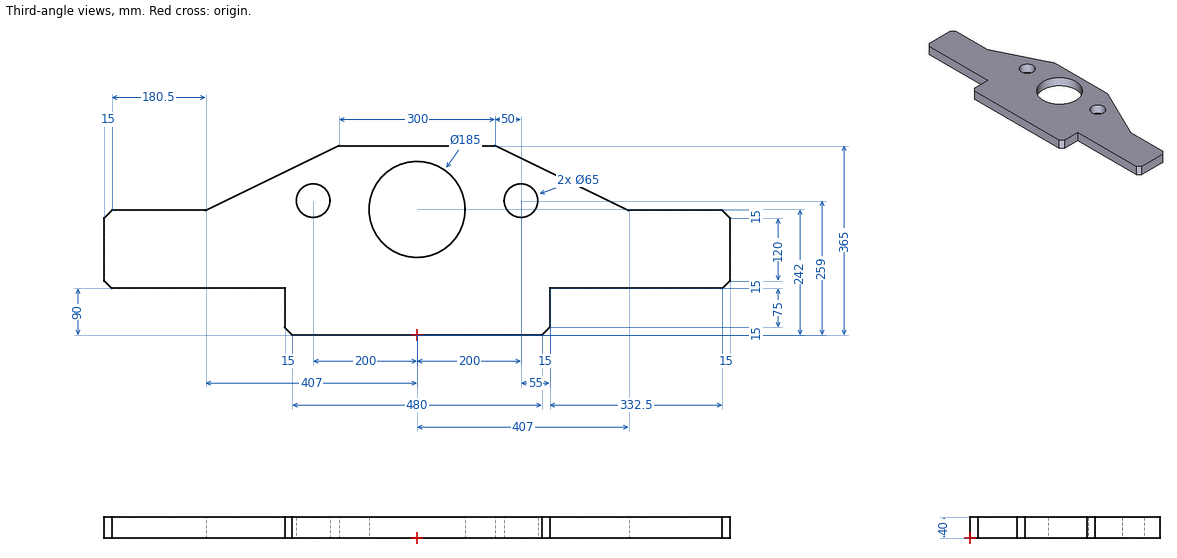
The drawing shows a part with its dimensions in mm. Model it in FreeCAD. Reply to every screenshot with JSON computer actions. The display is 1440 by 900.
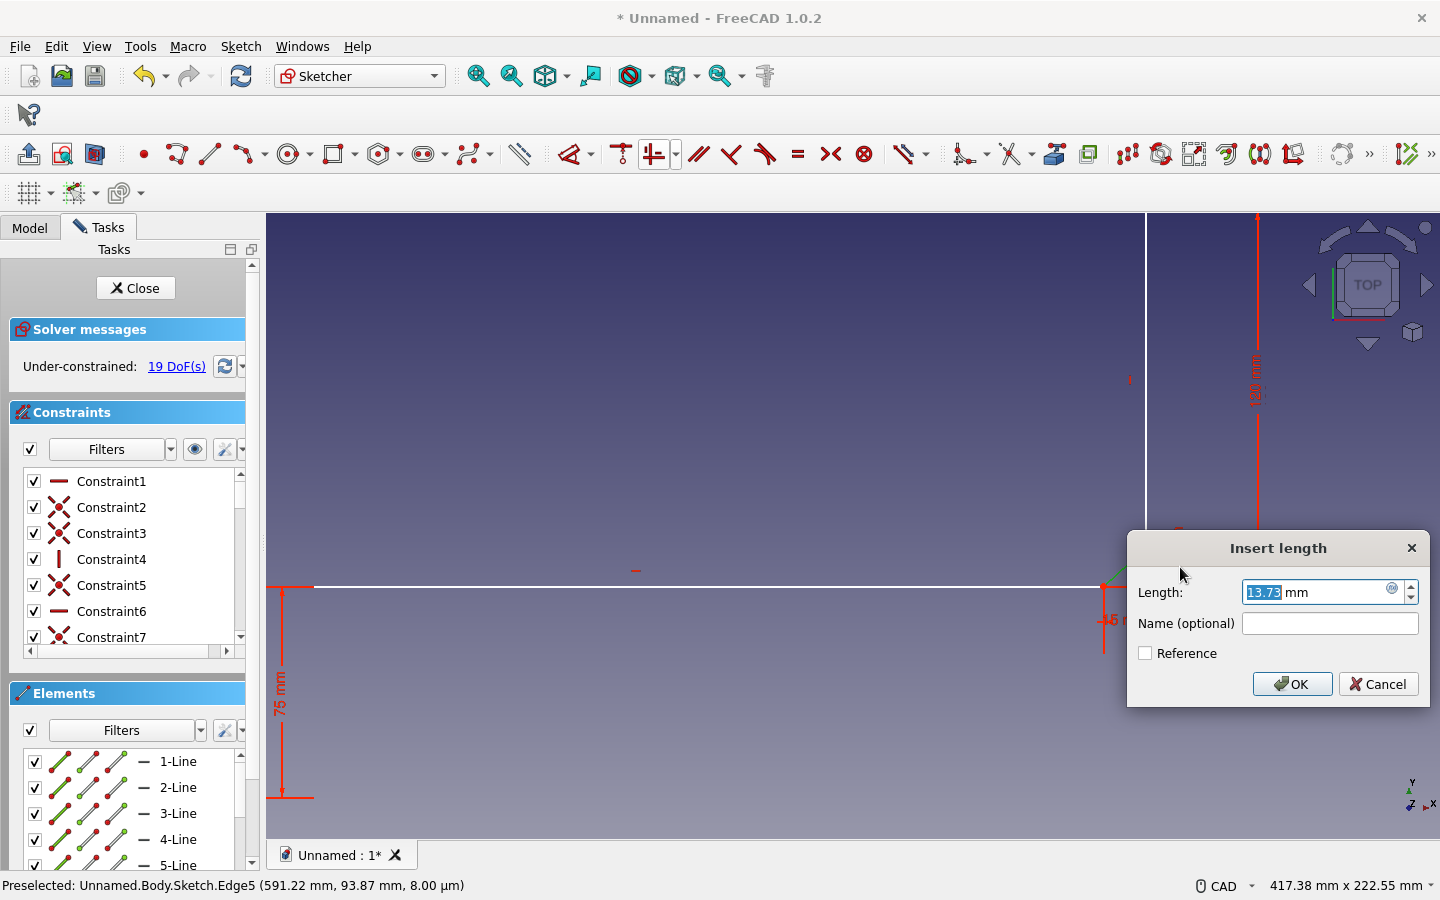
{"action": "type", "text": "15"}
{"action": "key", "text": "Return"}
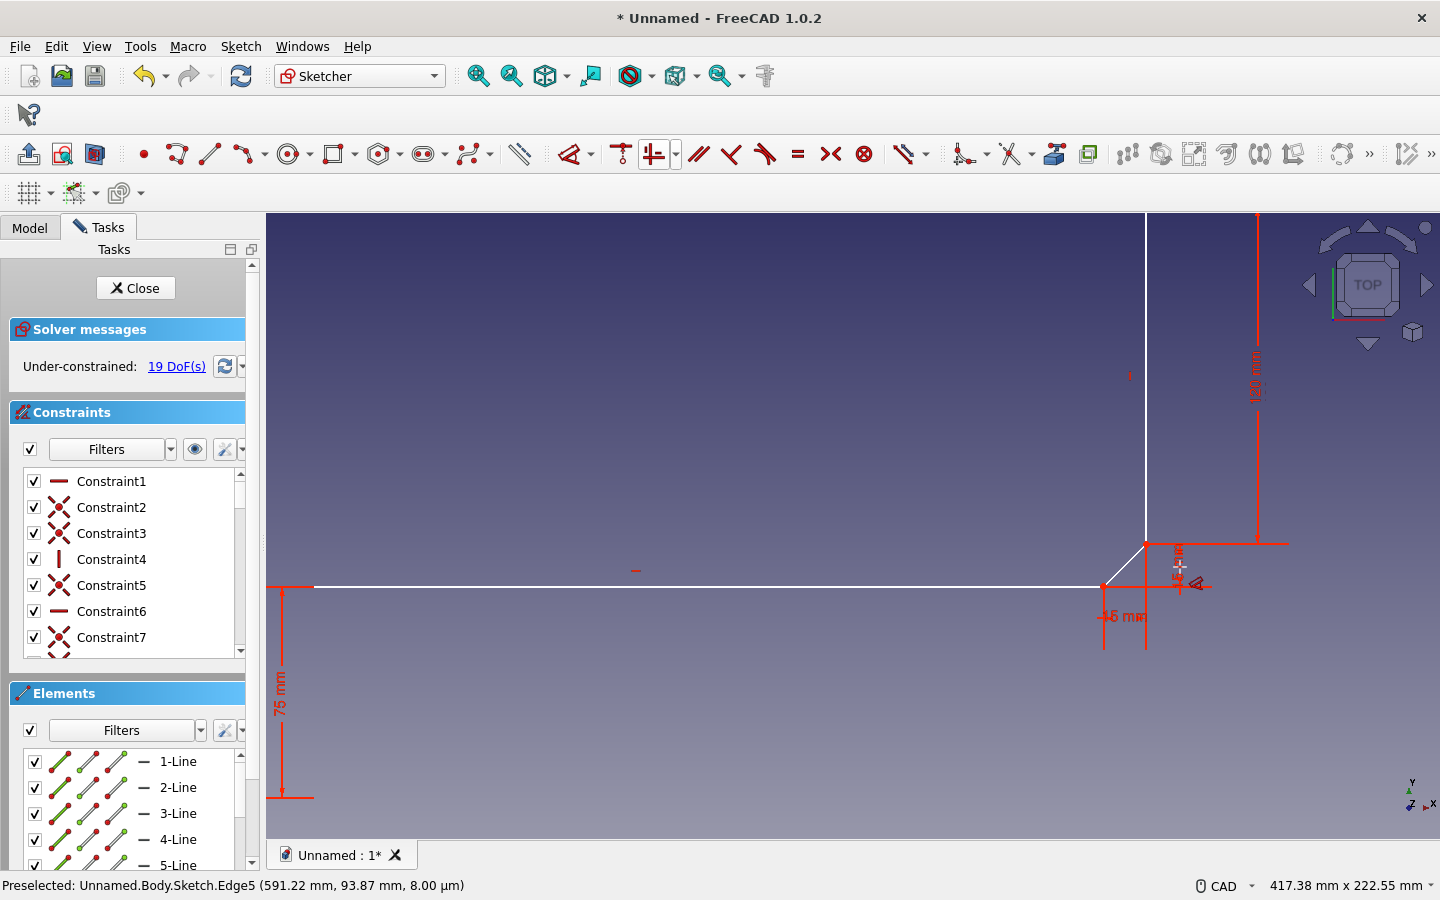
{"action": "scroll", "coordinate": [1121, 576], "scroll_direction": "down", "scroll_amount": 8}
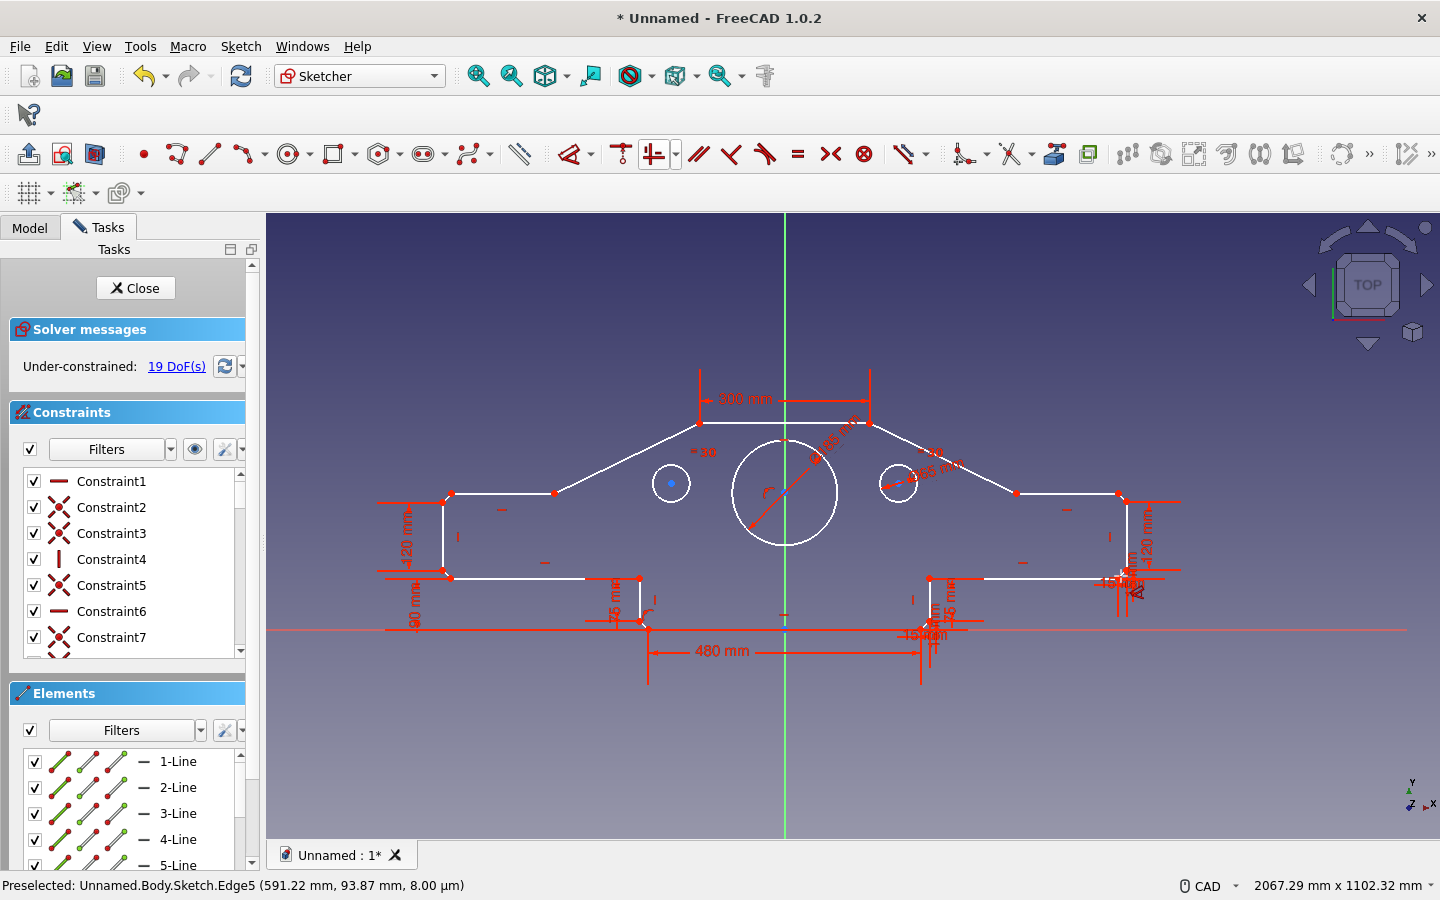
{"action": "scroll", "coordinate": [1124, 499], "scroll_direction": "up", "scroll_amount": 8}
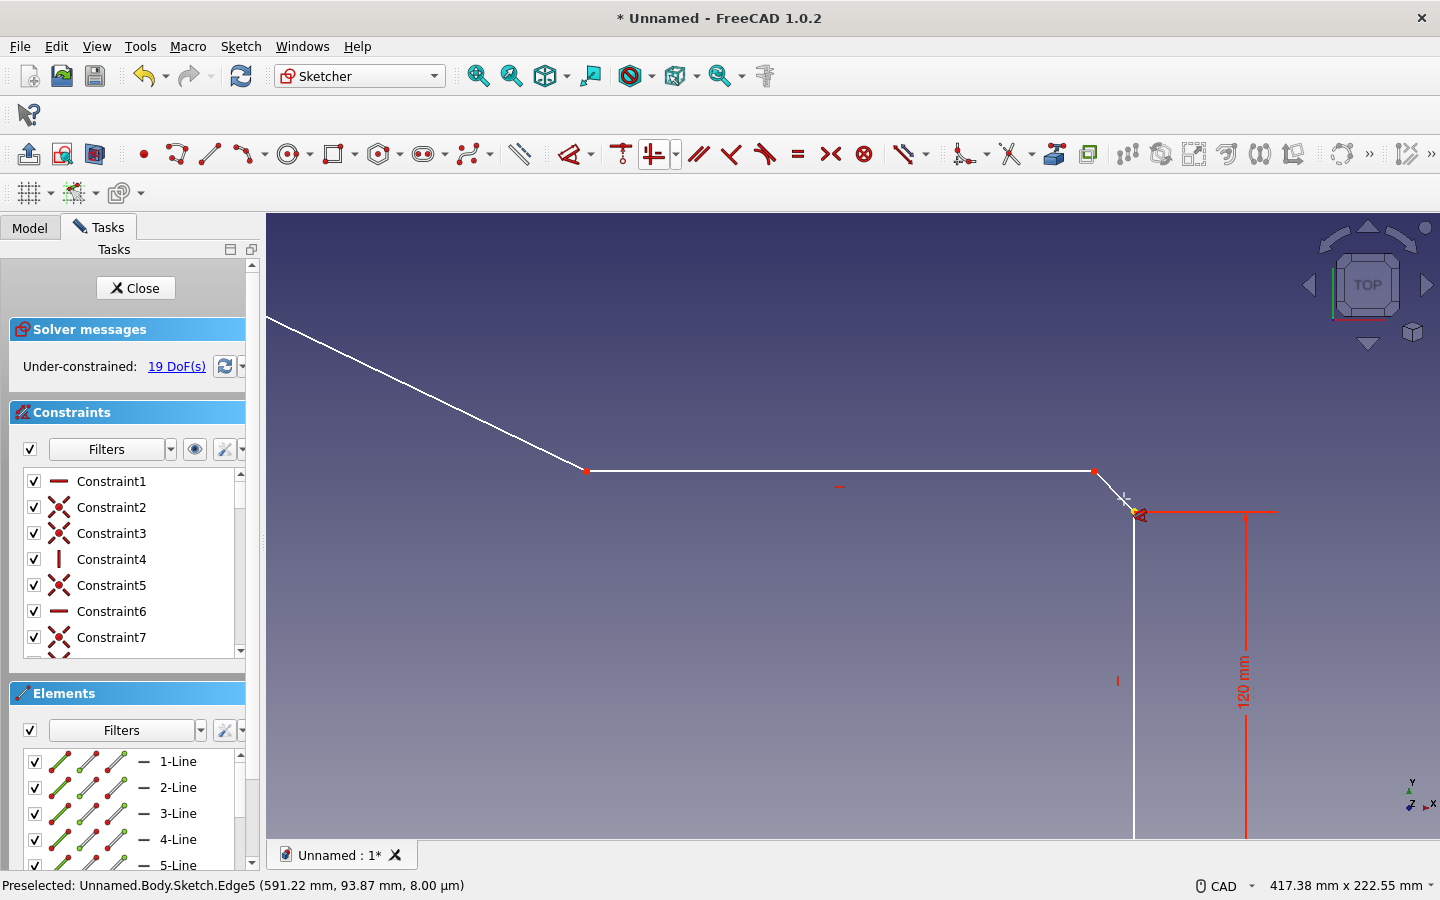
{"action": "left_click", "coordinate": [1122, 500]}
{"action": "left_click", "coordinate": [1114, 437]}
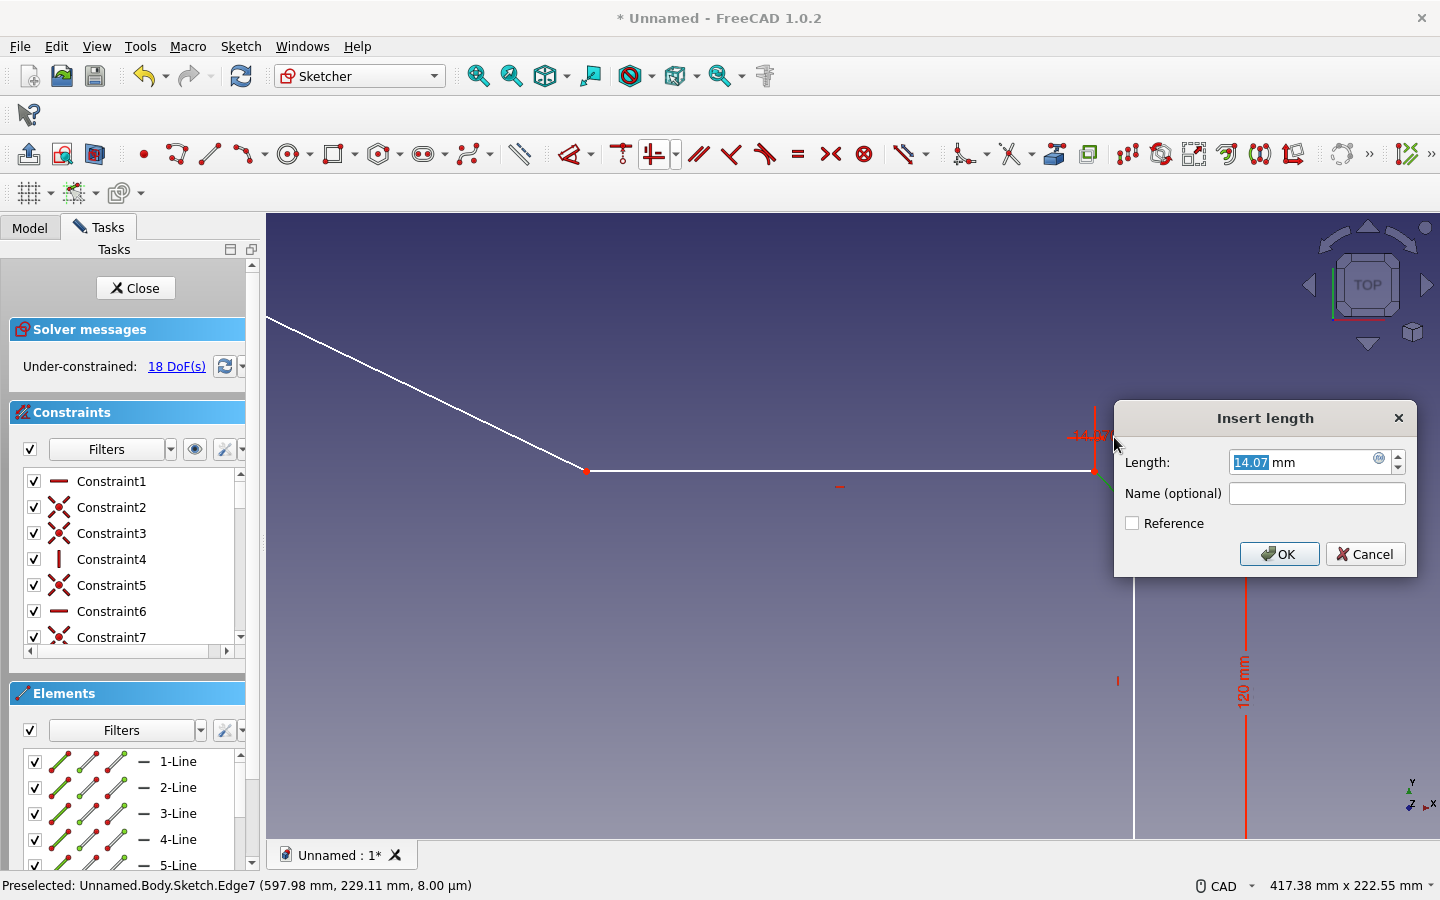
{"action": "type", "text": "15"}
{"action": "key", "text": "Return"}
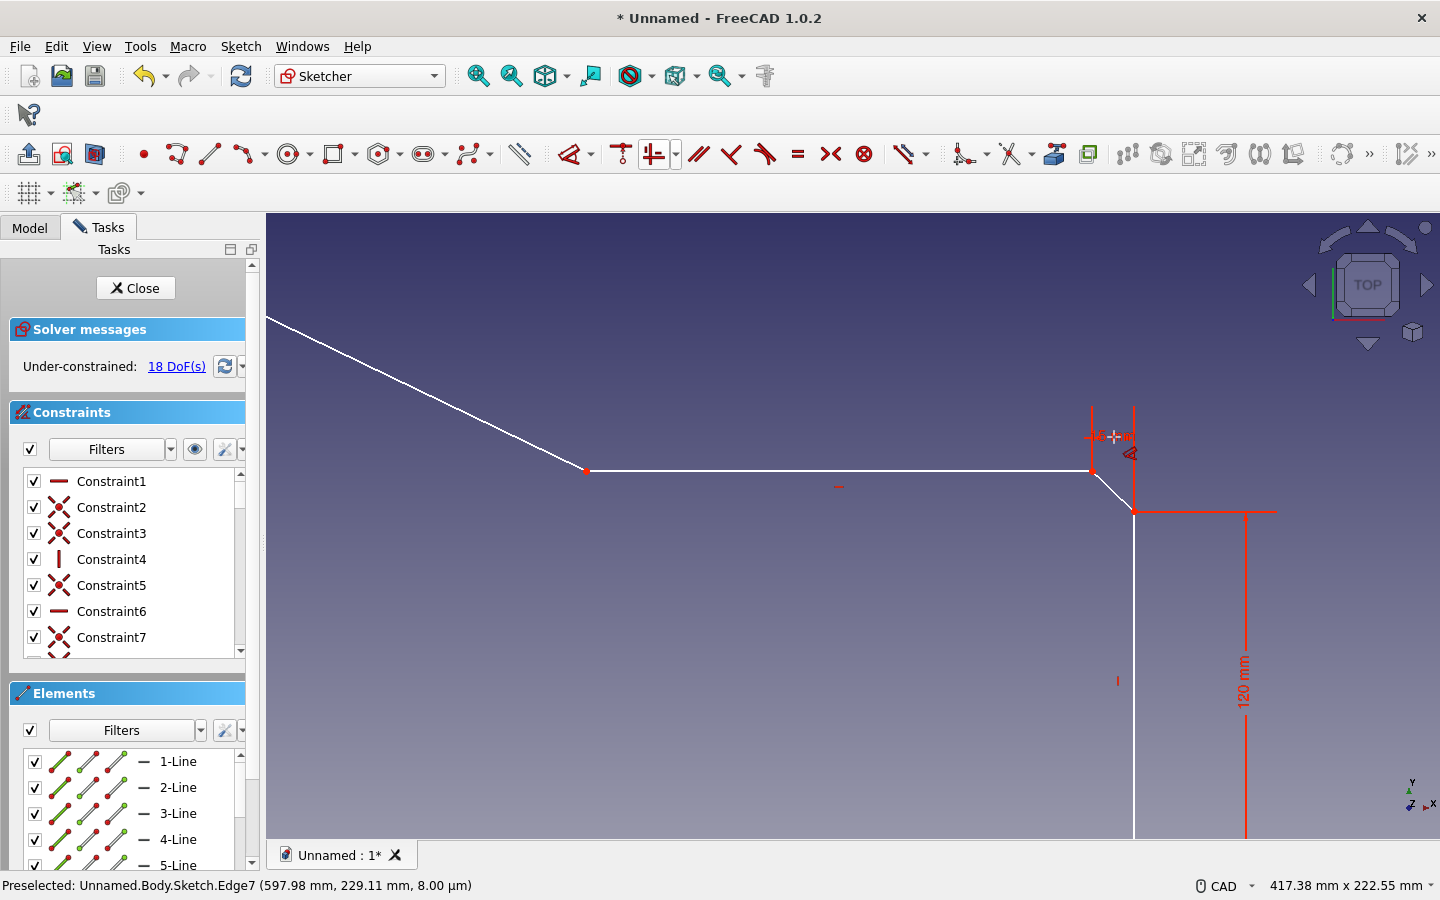
{"action": "left_click", "coordinate": [1122, 500]}
{"action": "left_click", "coordinate": [1168, 491]}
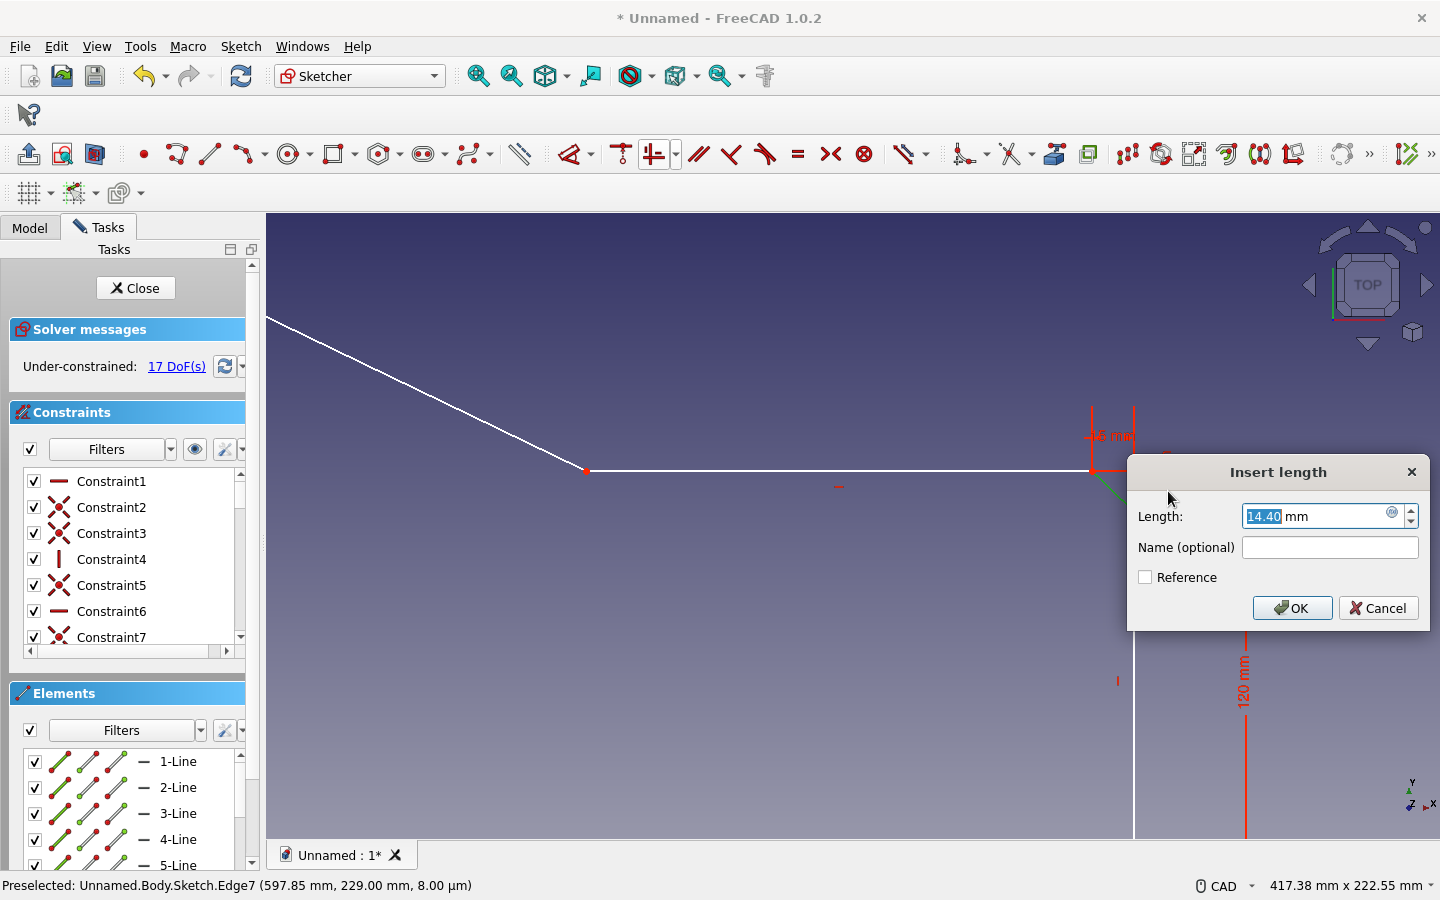
{"action": "type", "text": "15"}
{"action": "key", "text": "Return"}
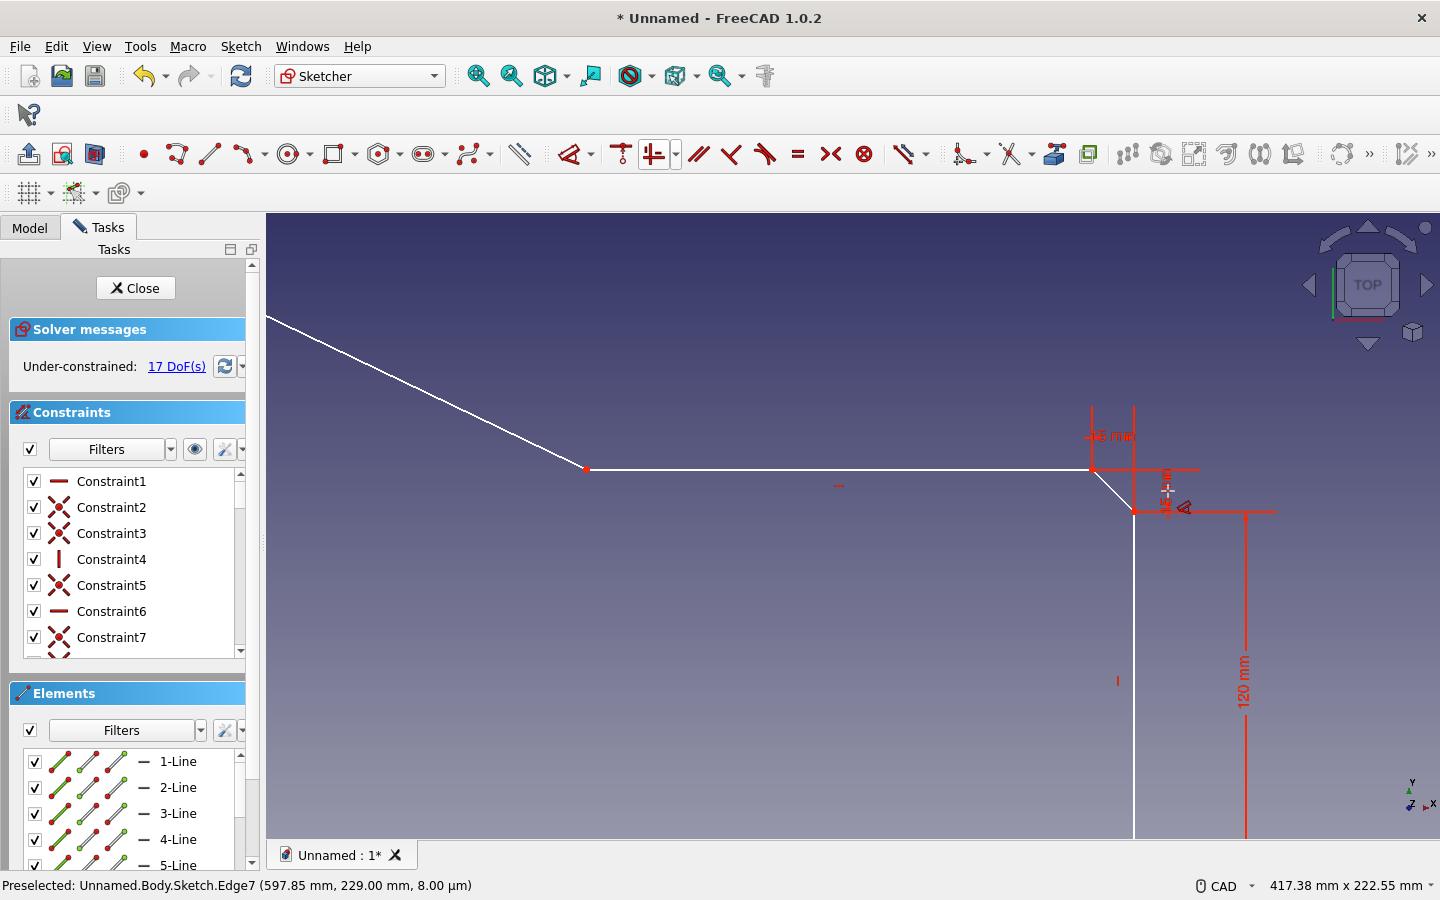
{"action": "scroll", "coordinate": [1124, 499], "scroll_direction": "down", "scroll_amount": 8}